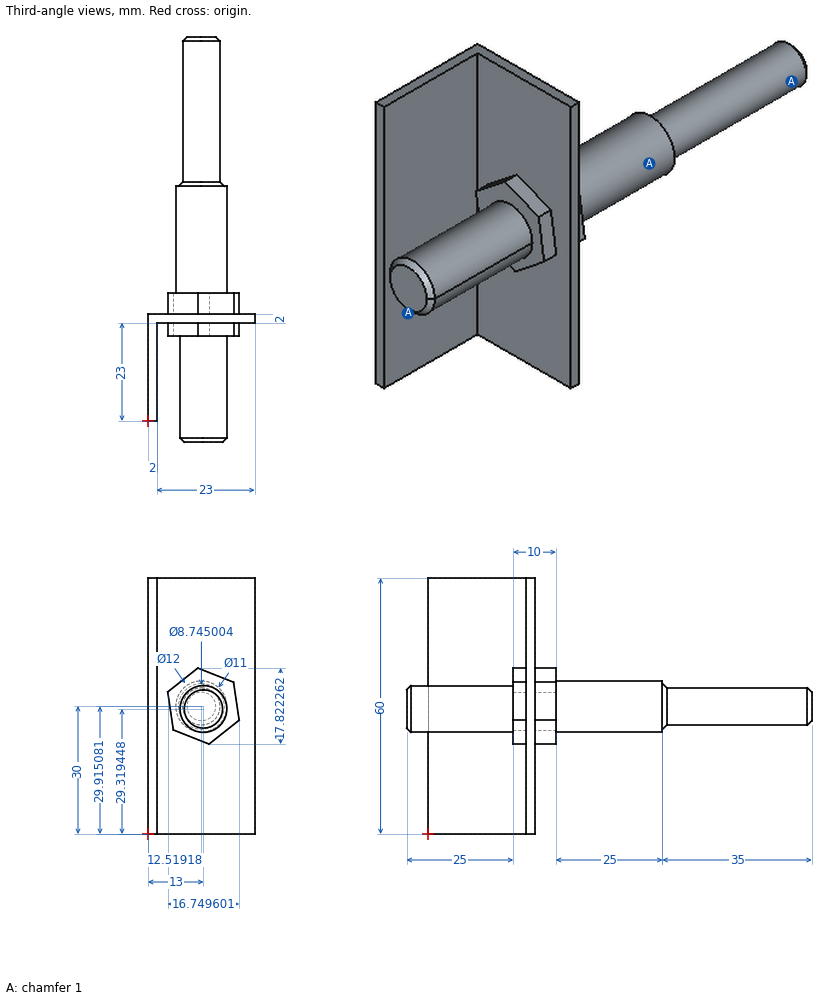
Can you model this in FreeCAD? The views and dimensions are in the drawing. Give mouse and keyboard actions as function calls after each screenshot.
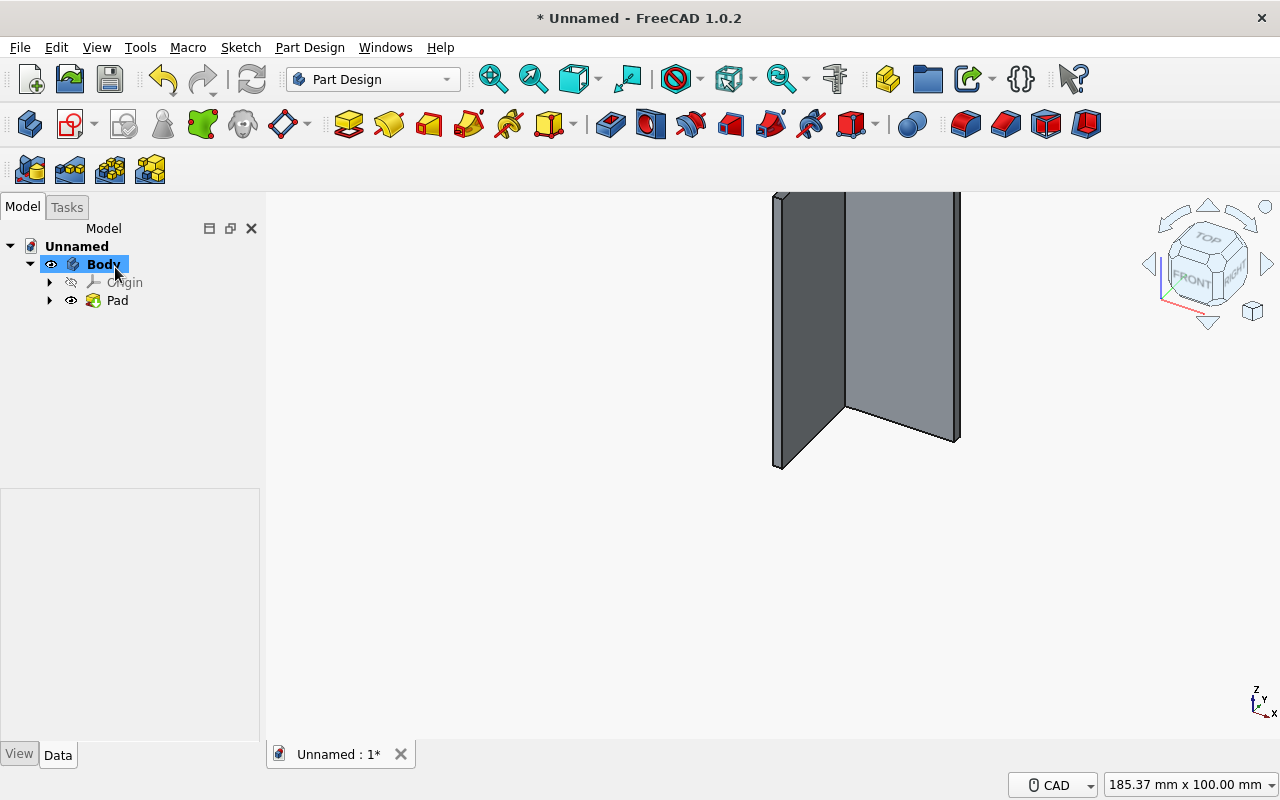
click(494, 80)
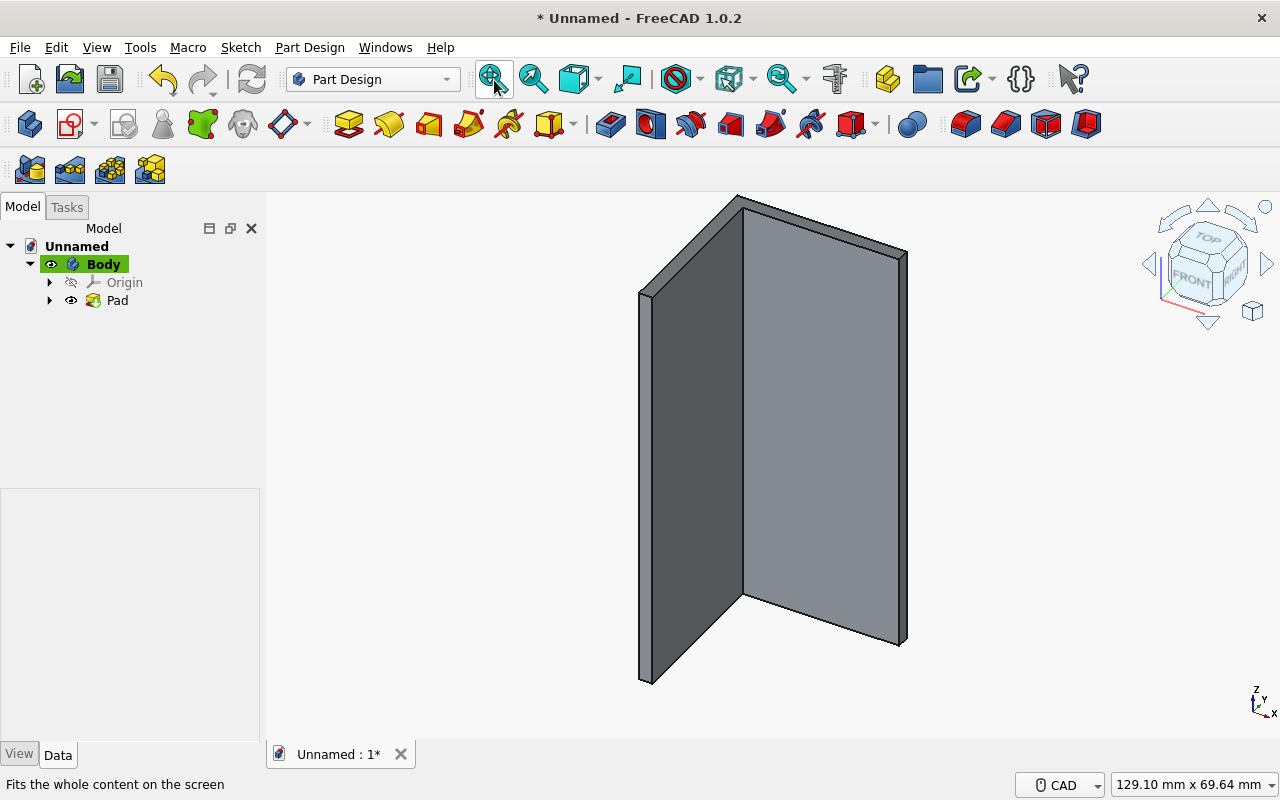
key(4)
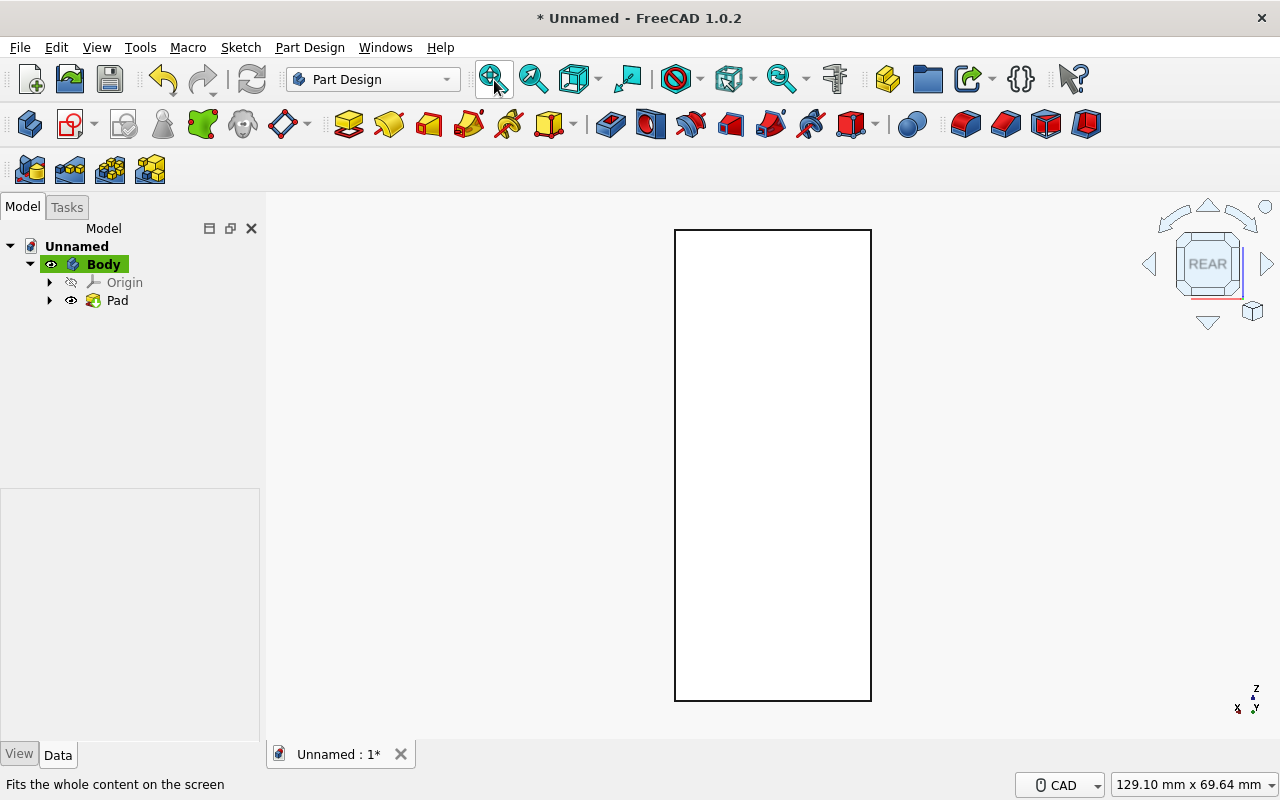
click(773, 330)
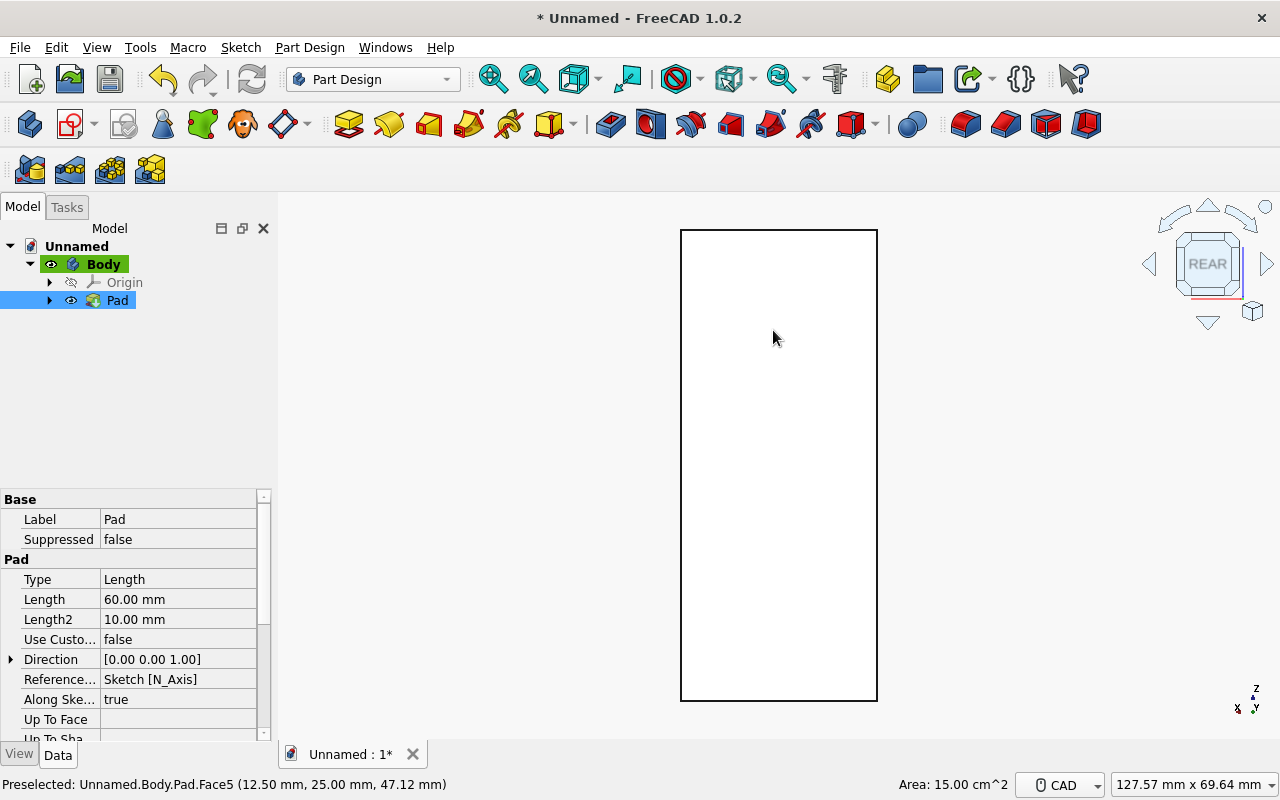
click(70, 124)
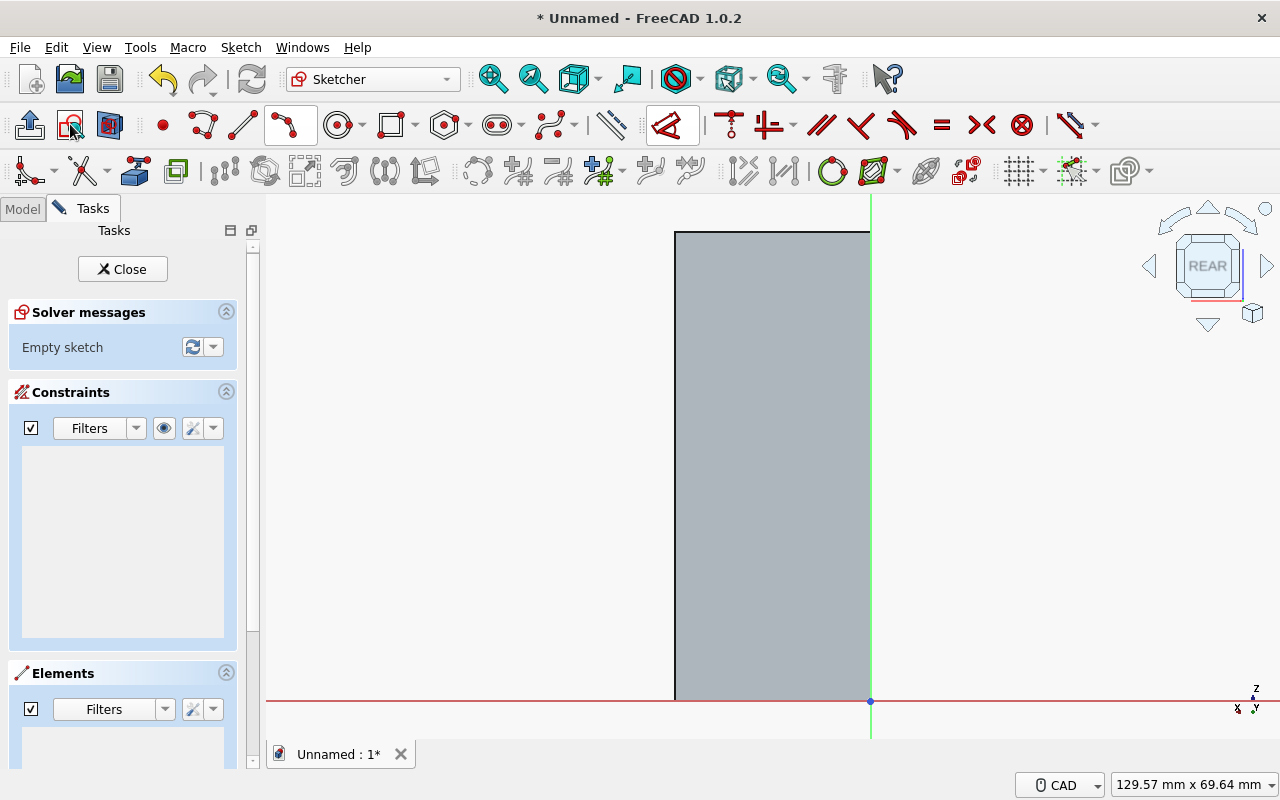
scroll(331, 222, down, 1)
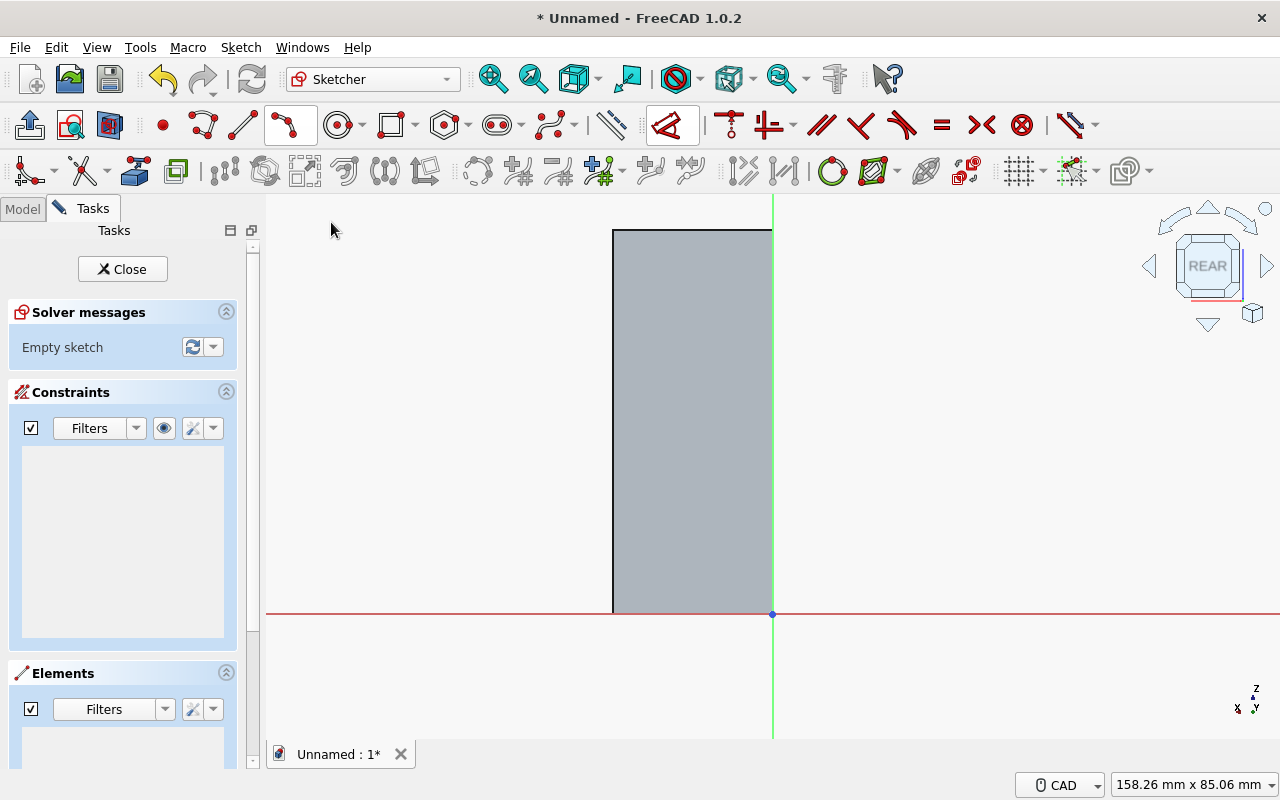
scroll(705, 537, up, 2)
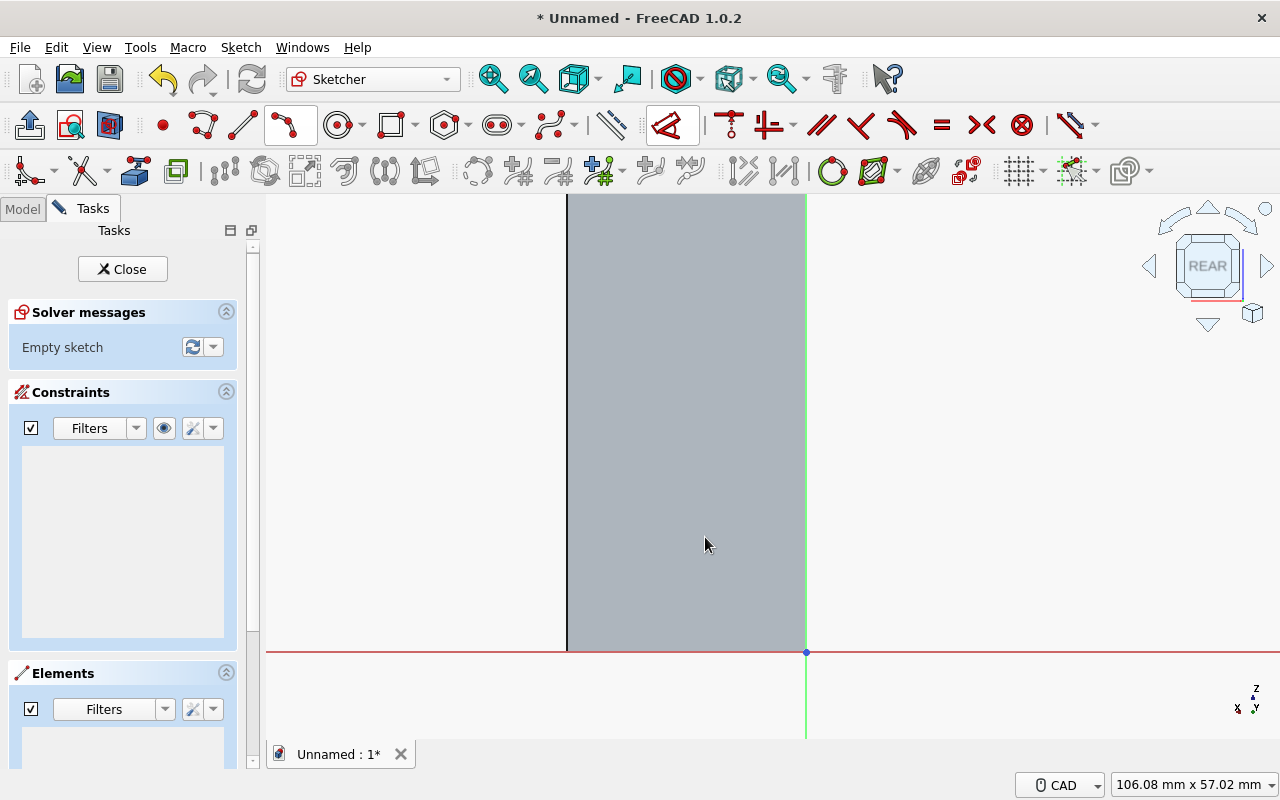
click(444, 126)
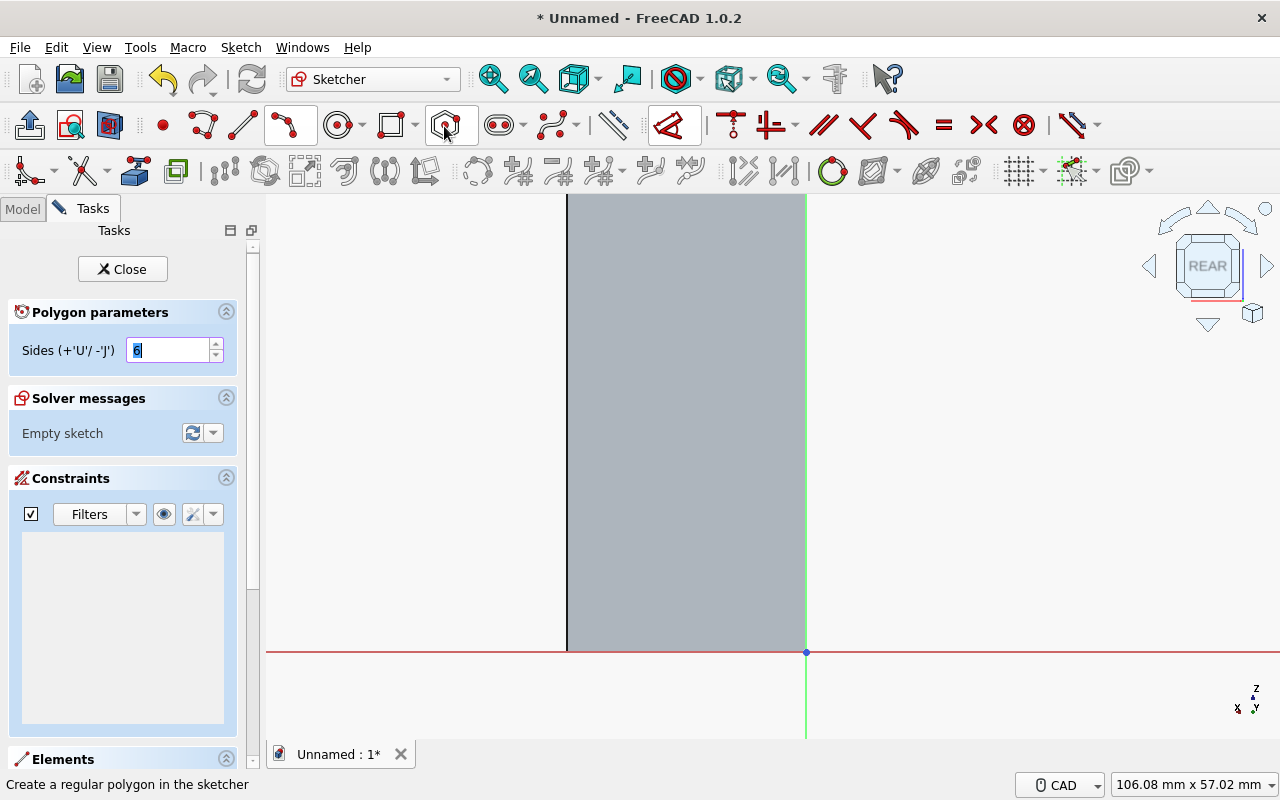
click(682, 365)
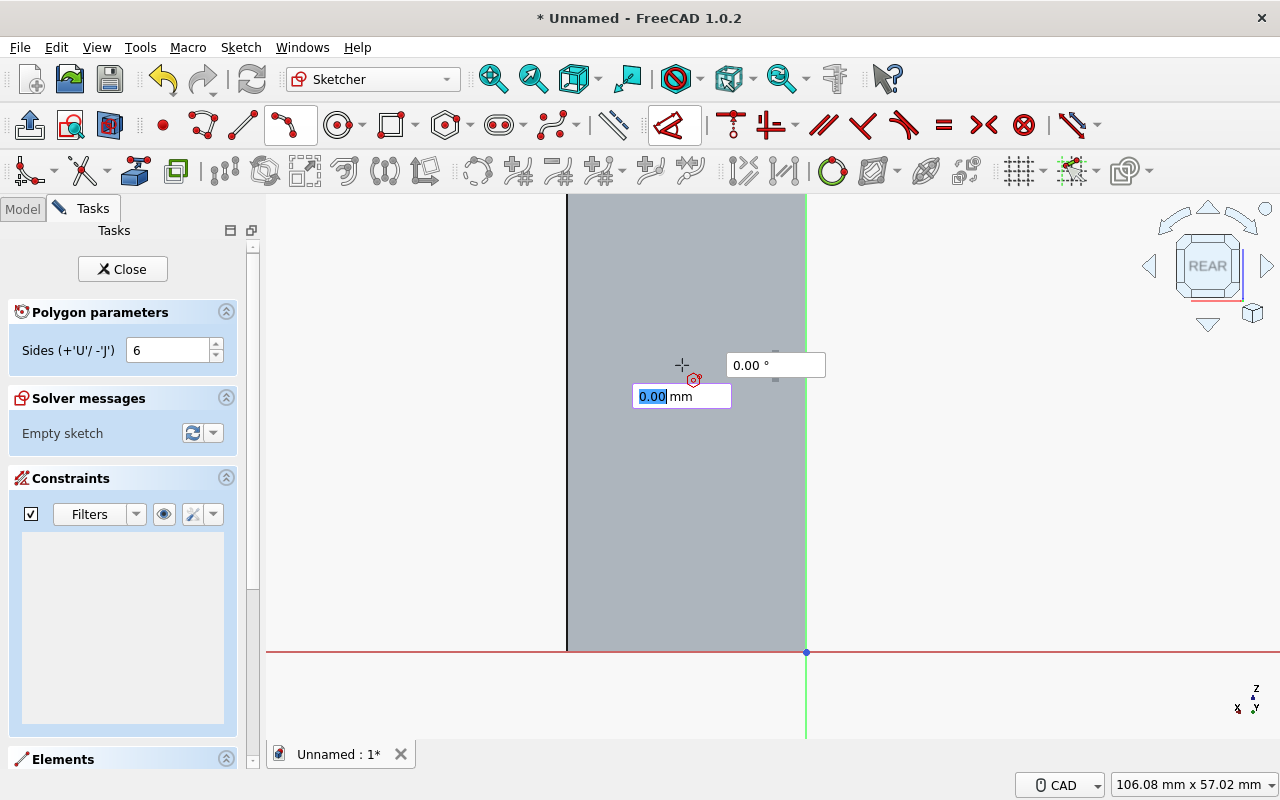
click(602, 397)
key(Escape)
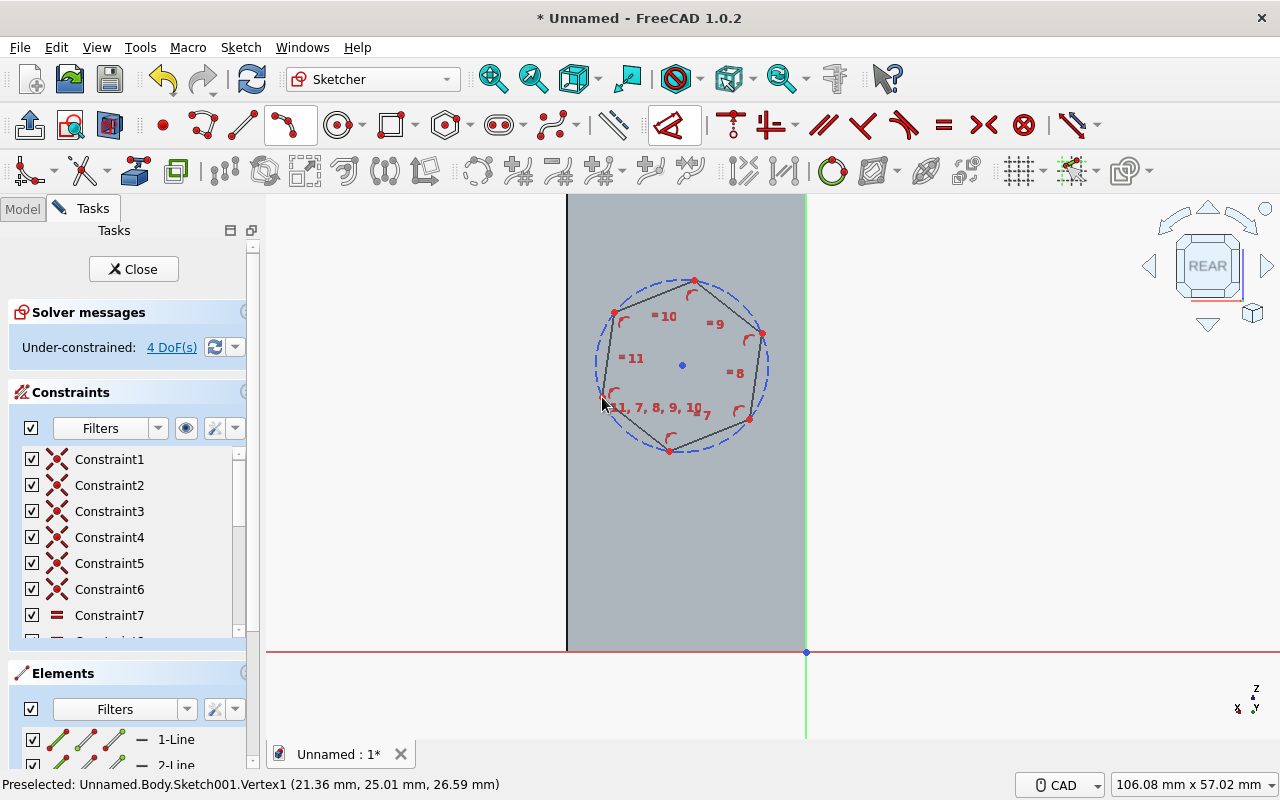
click(682, 366)